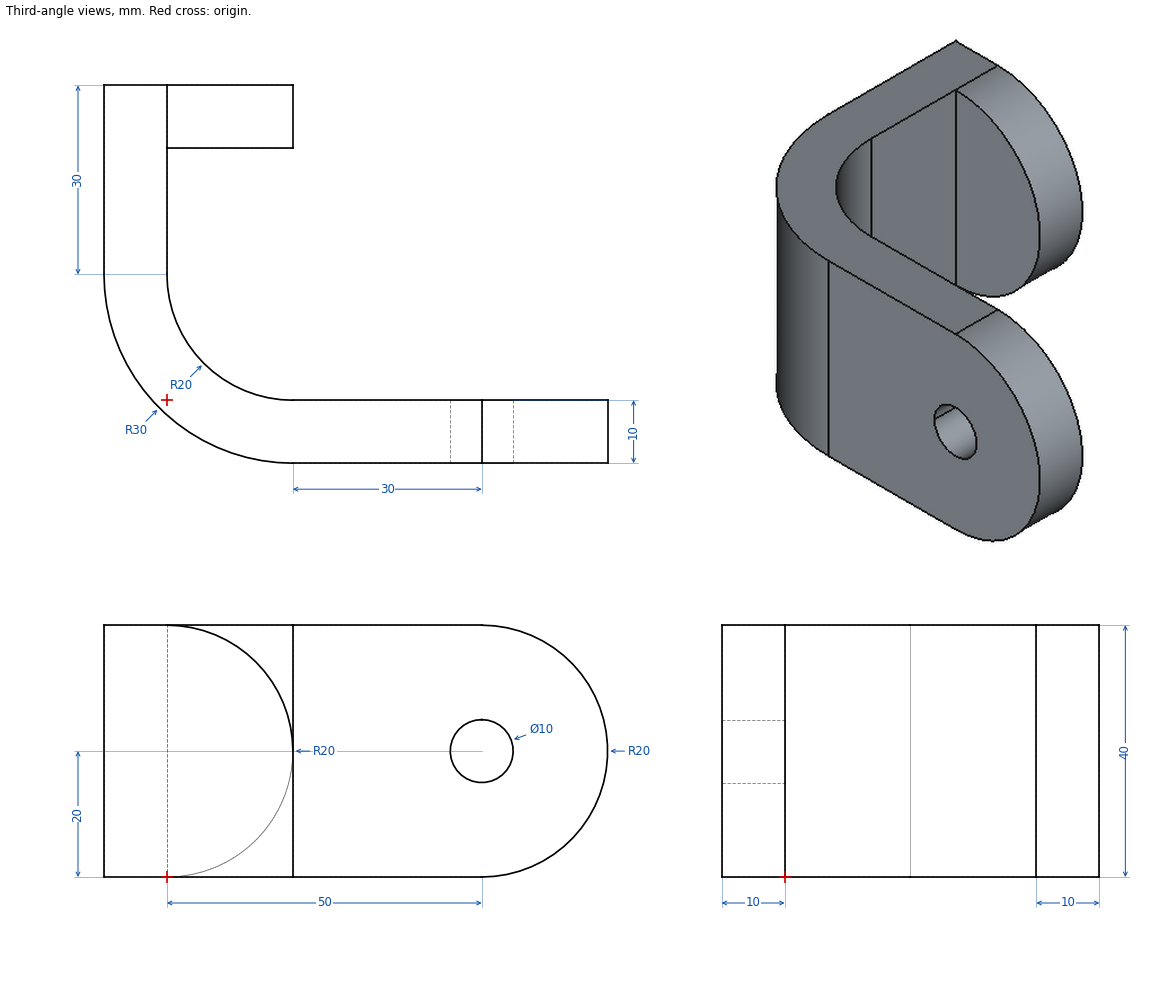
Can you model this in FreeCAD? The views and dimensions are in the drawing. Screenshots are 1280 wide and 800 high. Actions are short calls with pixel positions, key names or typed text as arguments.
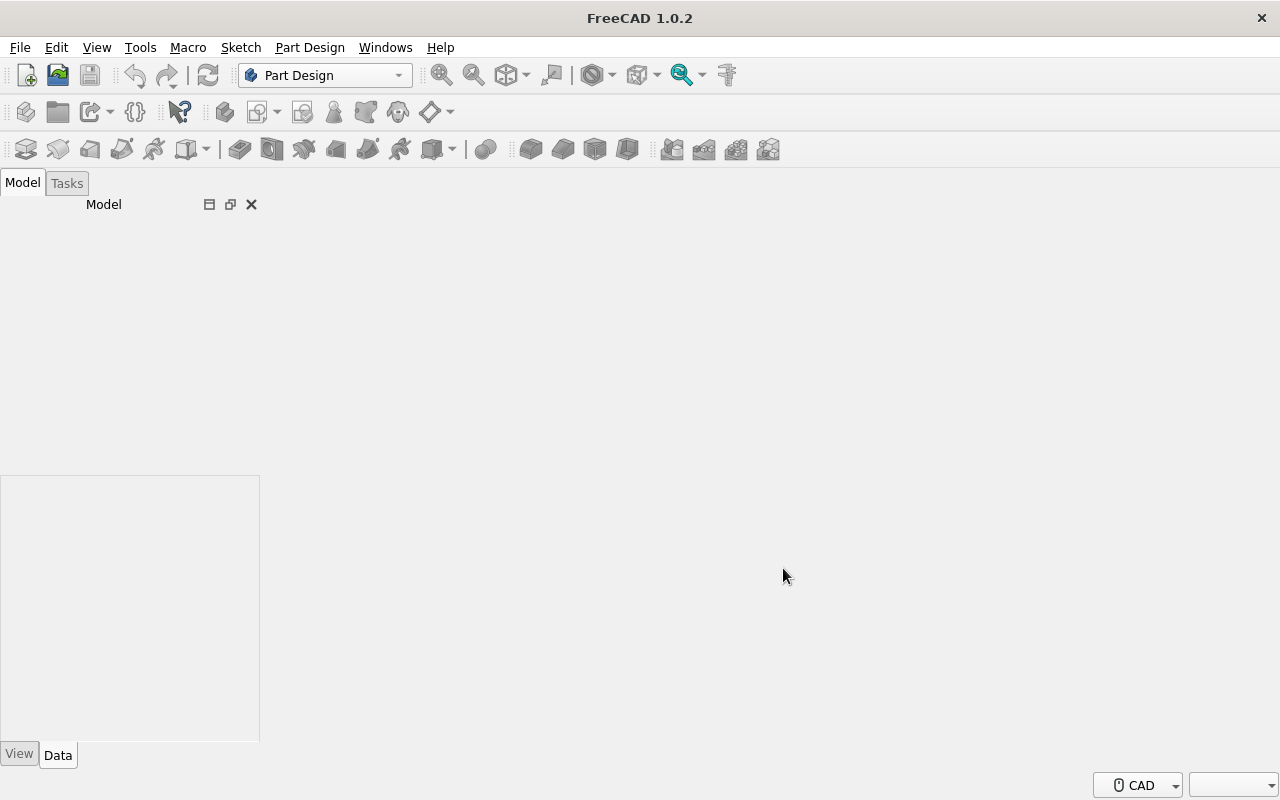
key(ctrl+n)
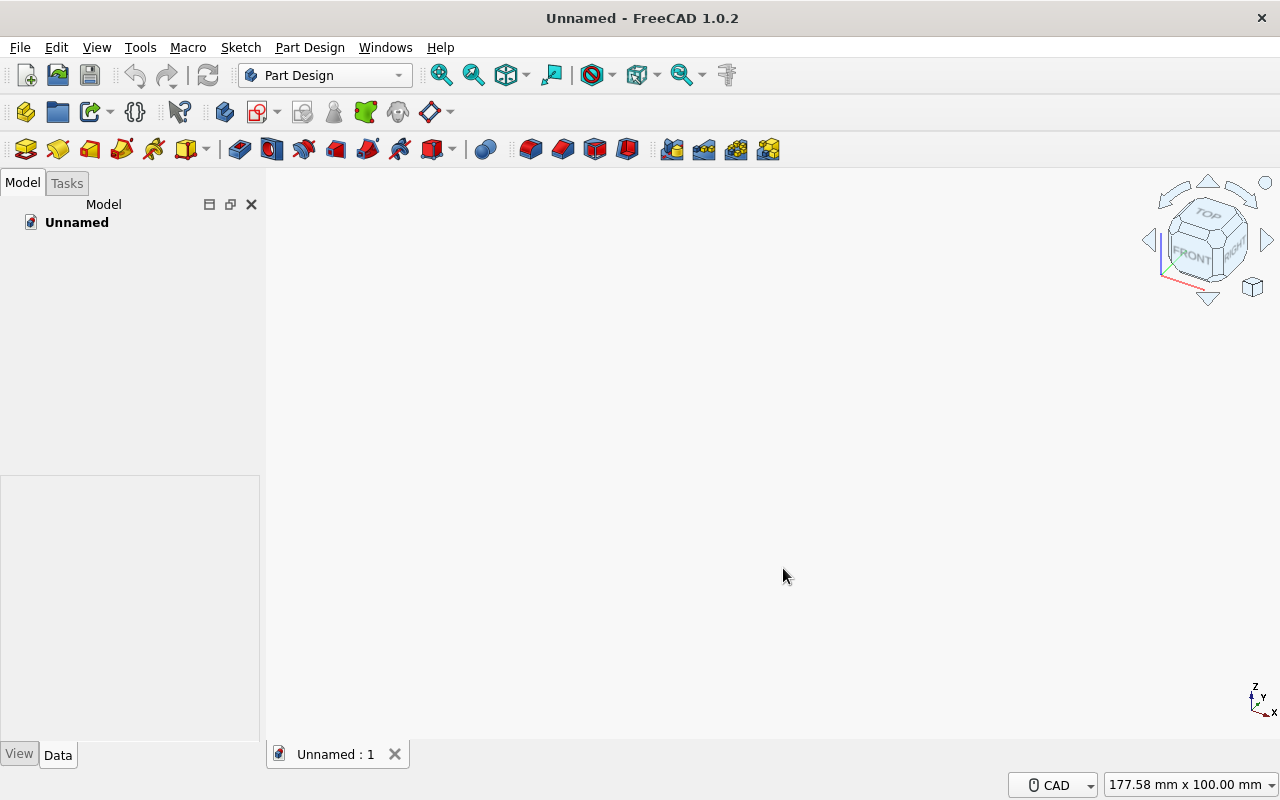
click(258, 112)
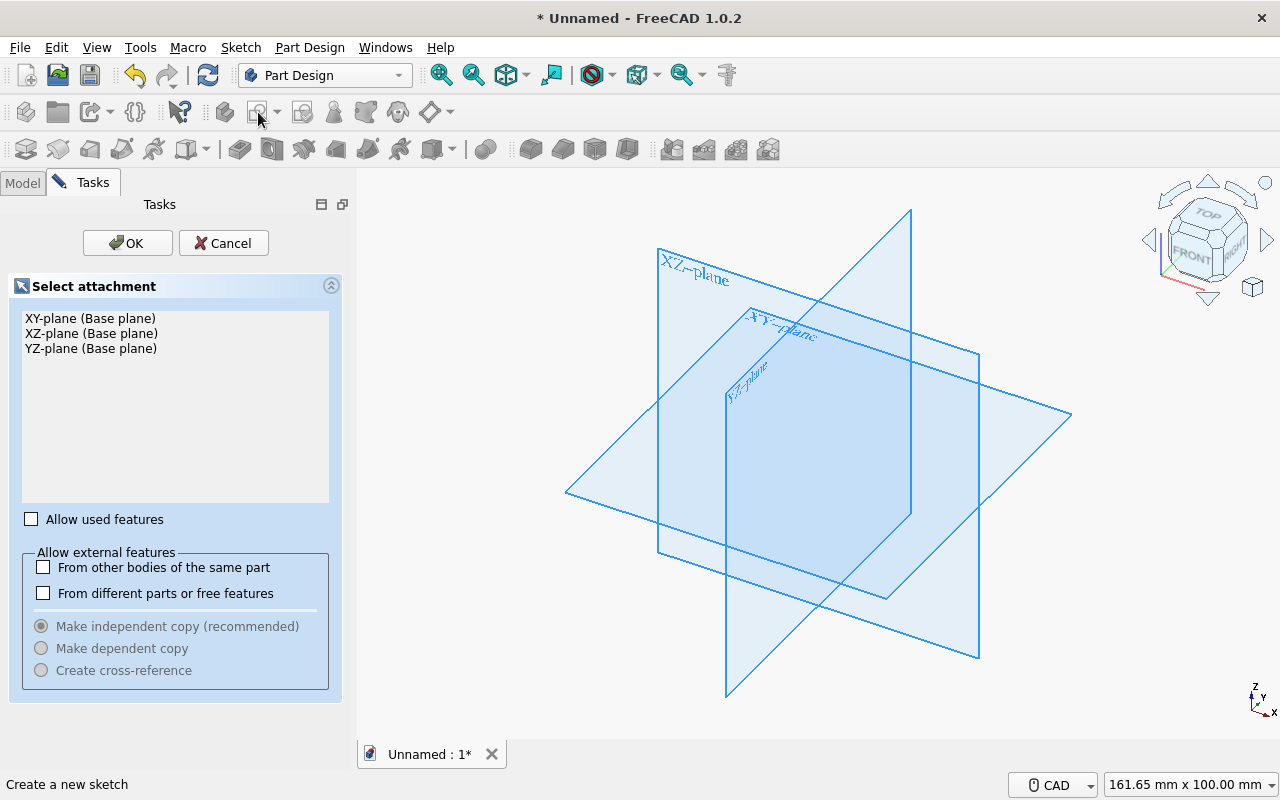
click(82, 318)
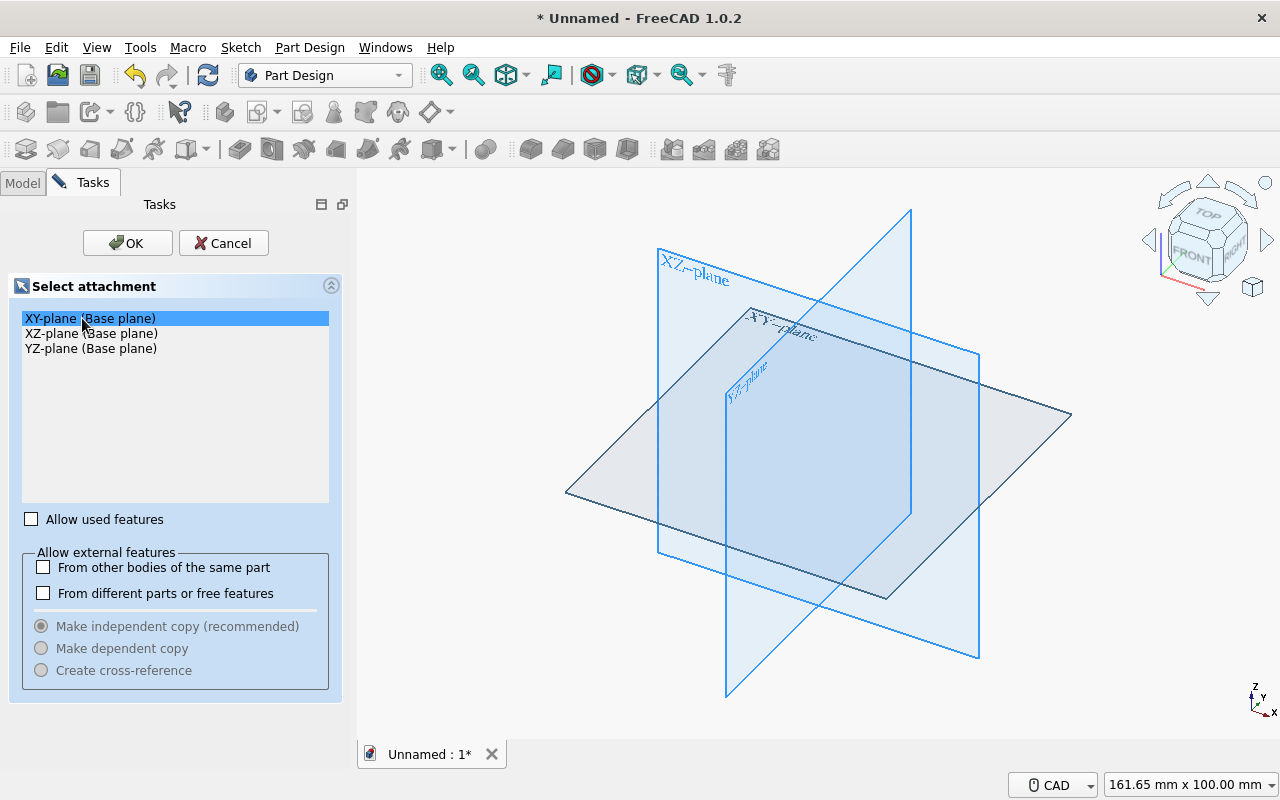
click(128, 243)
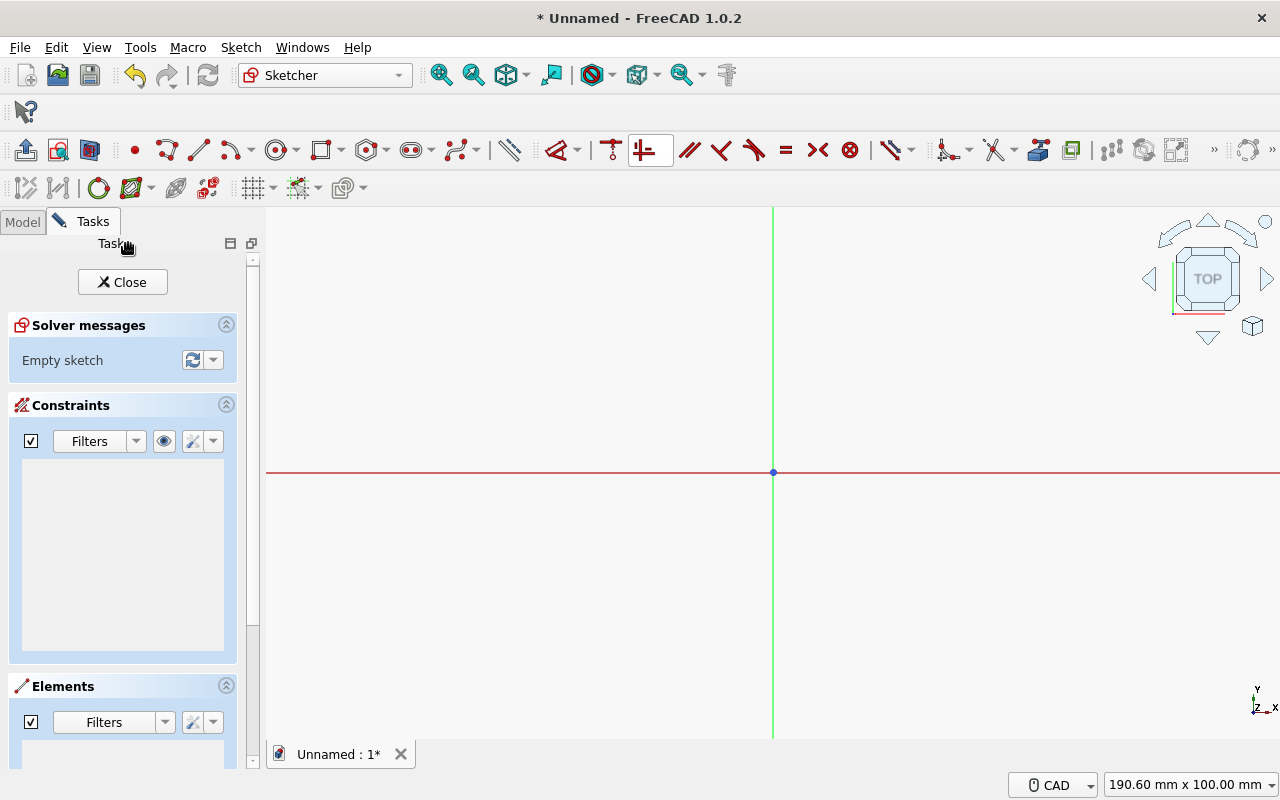
scroll(294, 711, down, 1)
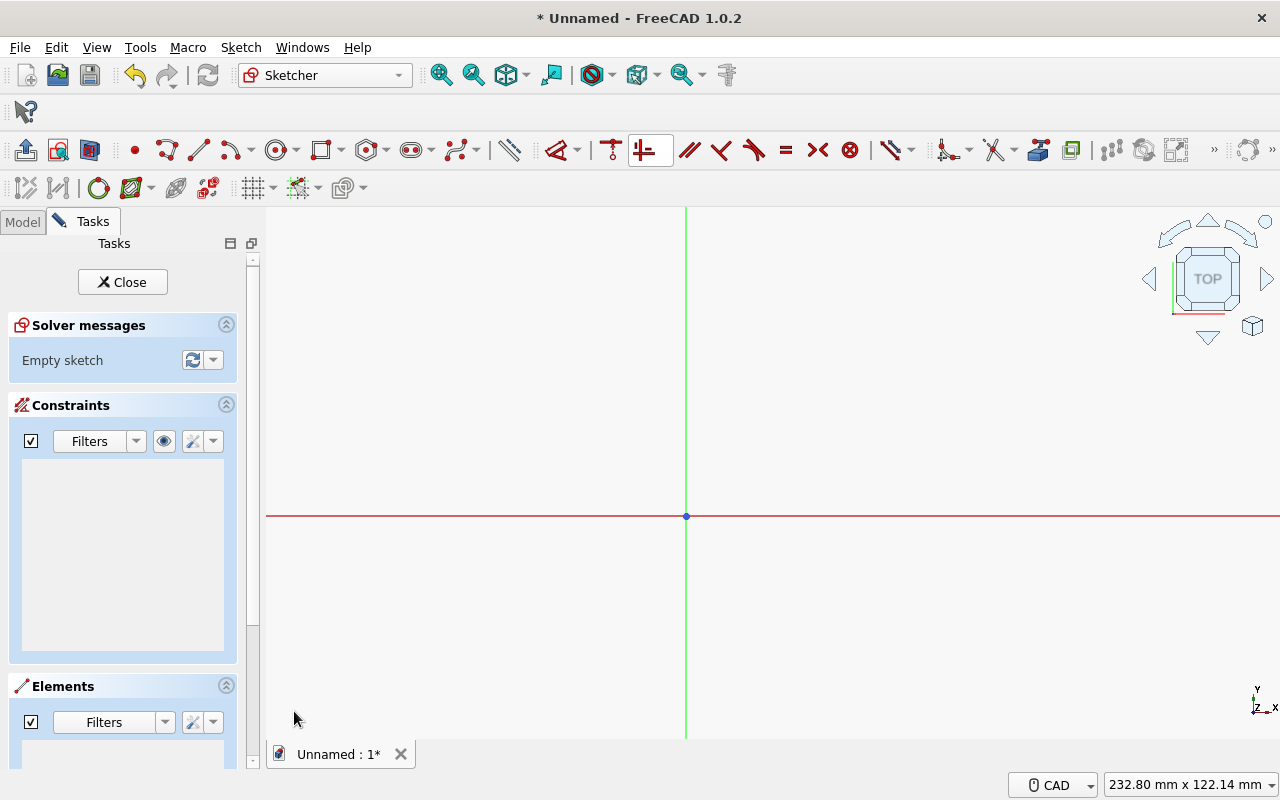
click(168, 150)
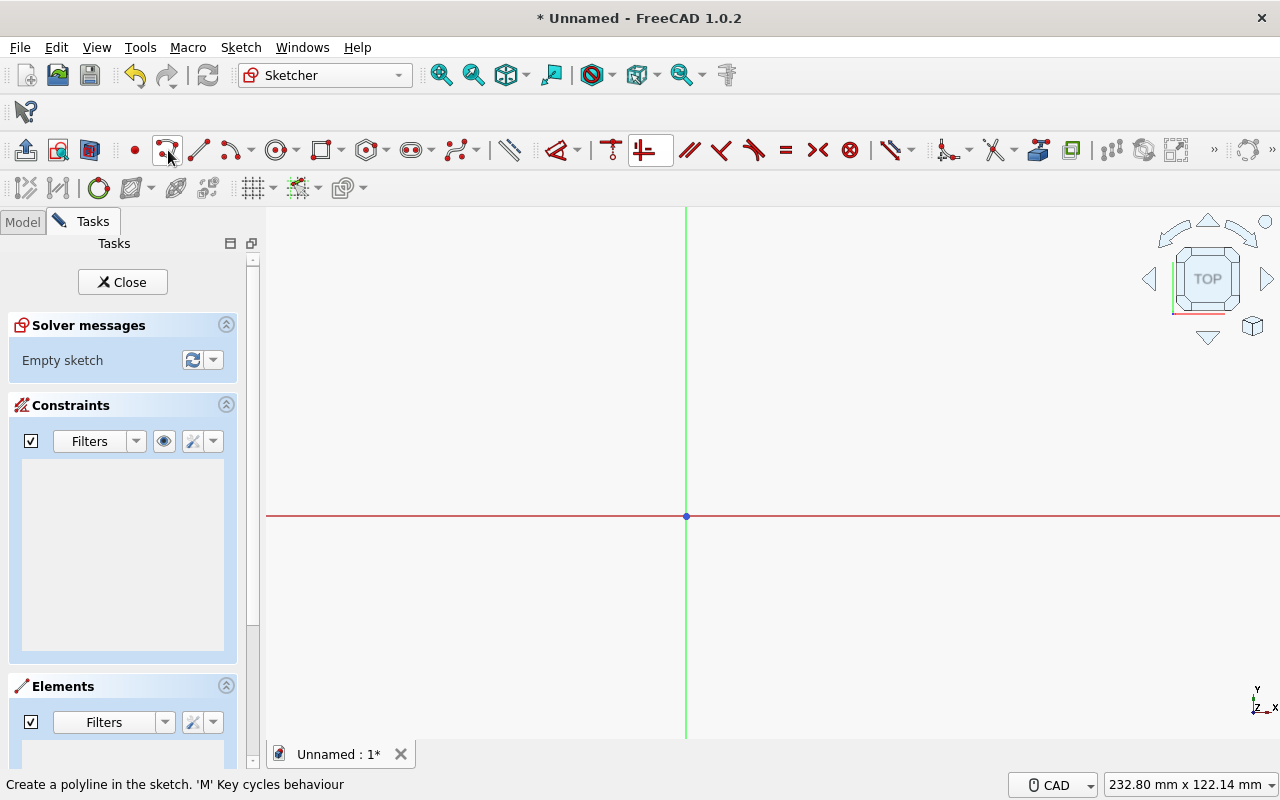
click(686, 429)
click(695, 299)
click(643, 299)
click(643, 429)
right_click(643, 429)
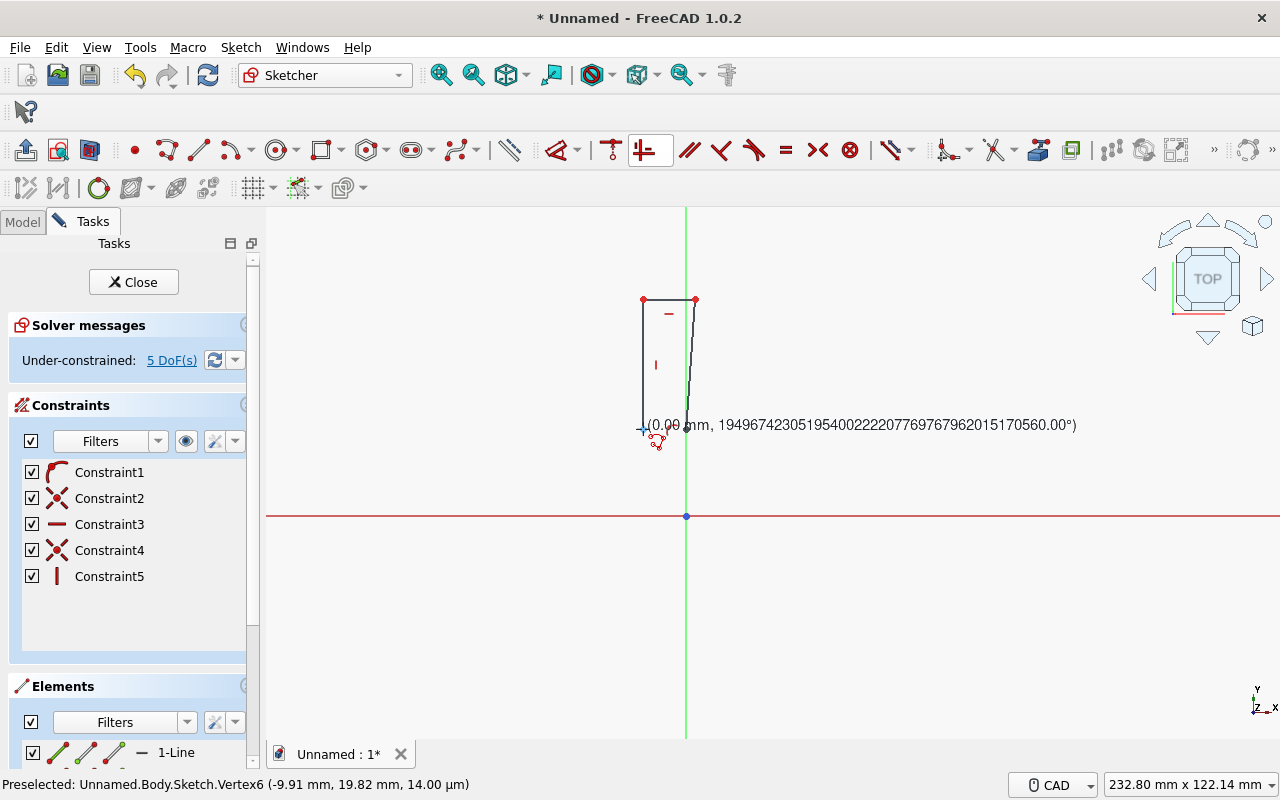
click(773, 560)
click(904, 560)
click(904, 516)
click(773, 507)
right_click(773, 507)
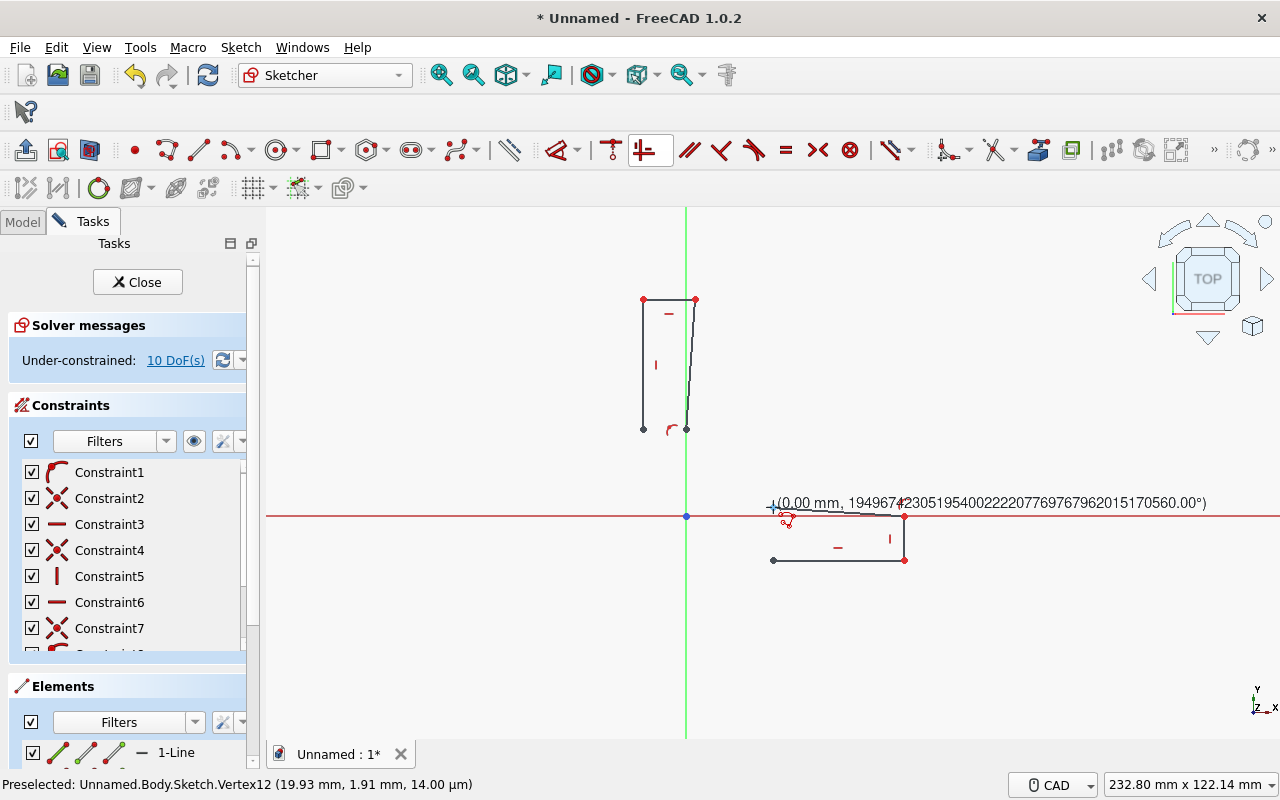
key(g)
key(3)
key(a)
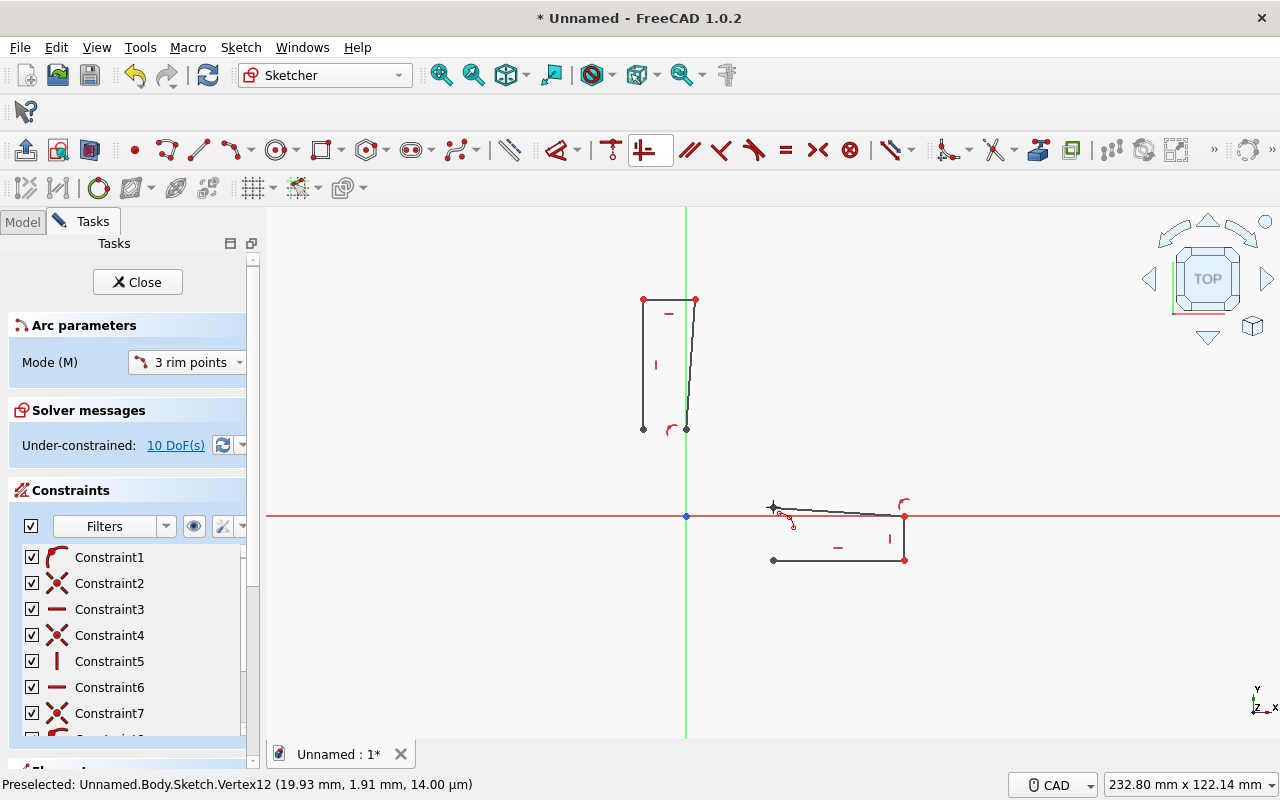
click(643, 430)
click(773, 561)
click(657, 489)